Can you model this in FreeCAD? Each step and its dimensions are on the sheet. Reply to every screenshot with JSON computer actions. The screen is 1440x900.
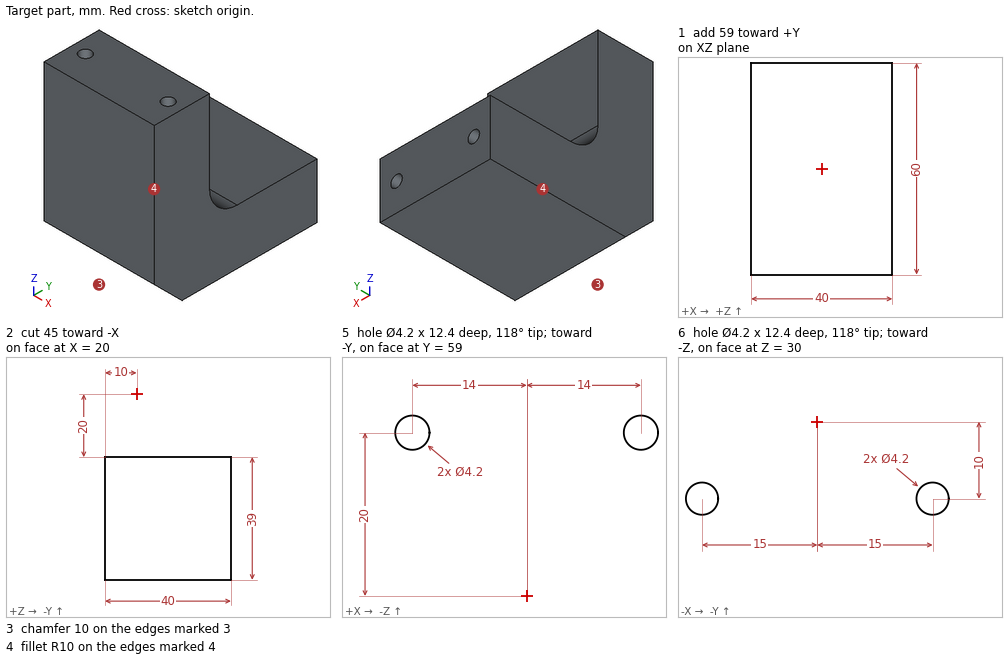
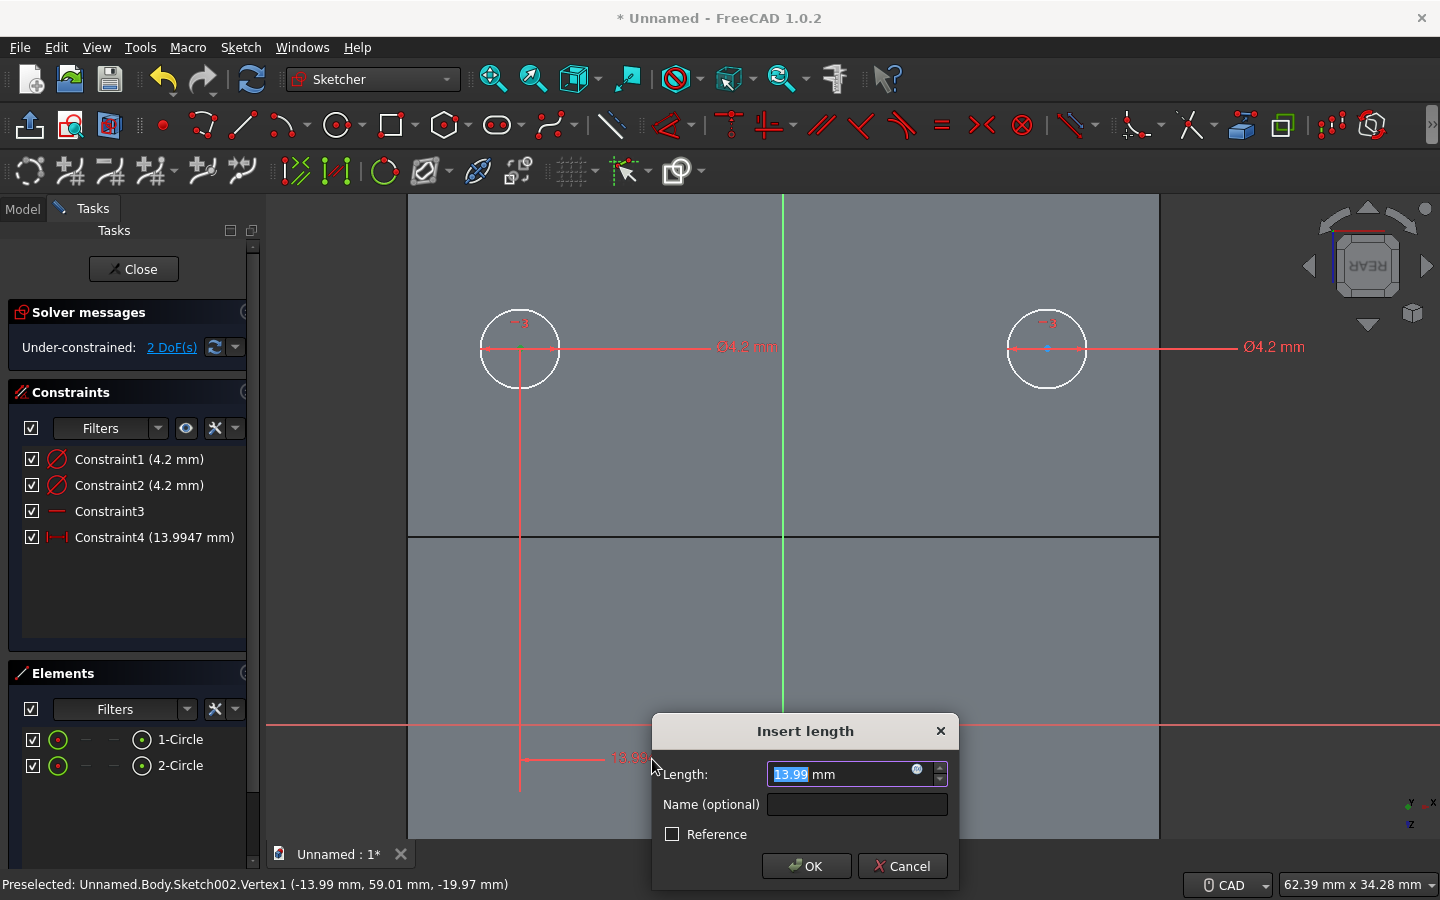
{"action": "type", "text": "14"}
{"action": "key", "text": "Return"}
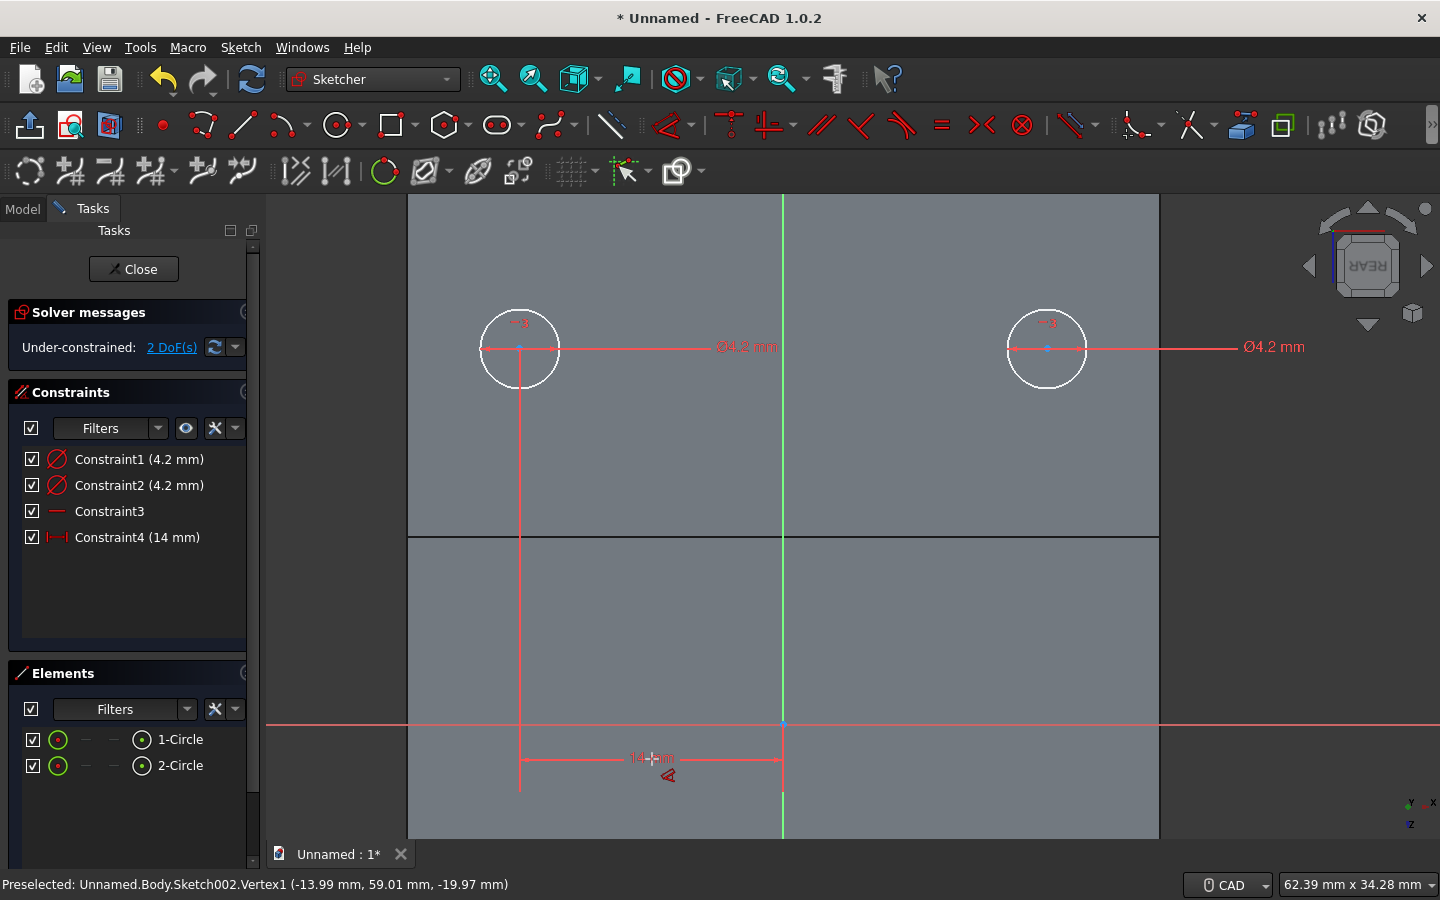
{"action": "left_click", "coordinate": [520, 349]}
{"action": "left_click", "coordinate": [486, 537]}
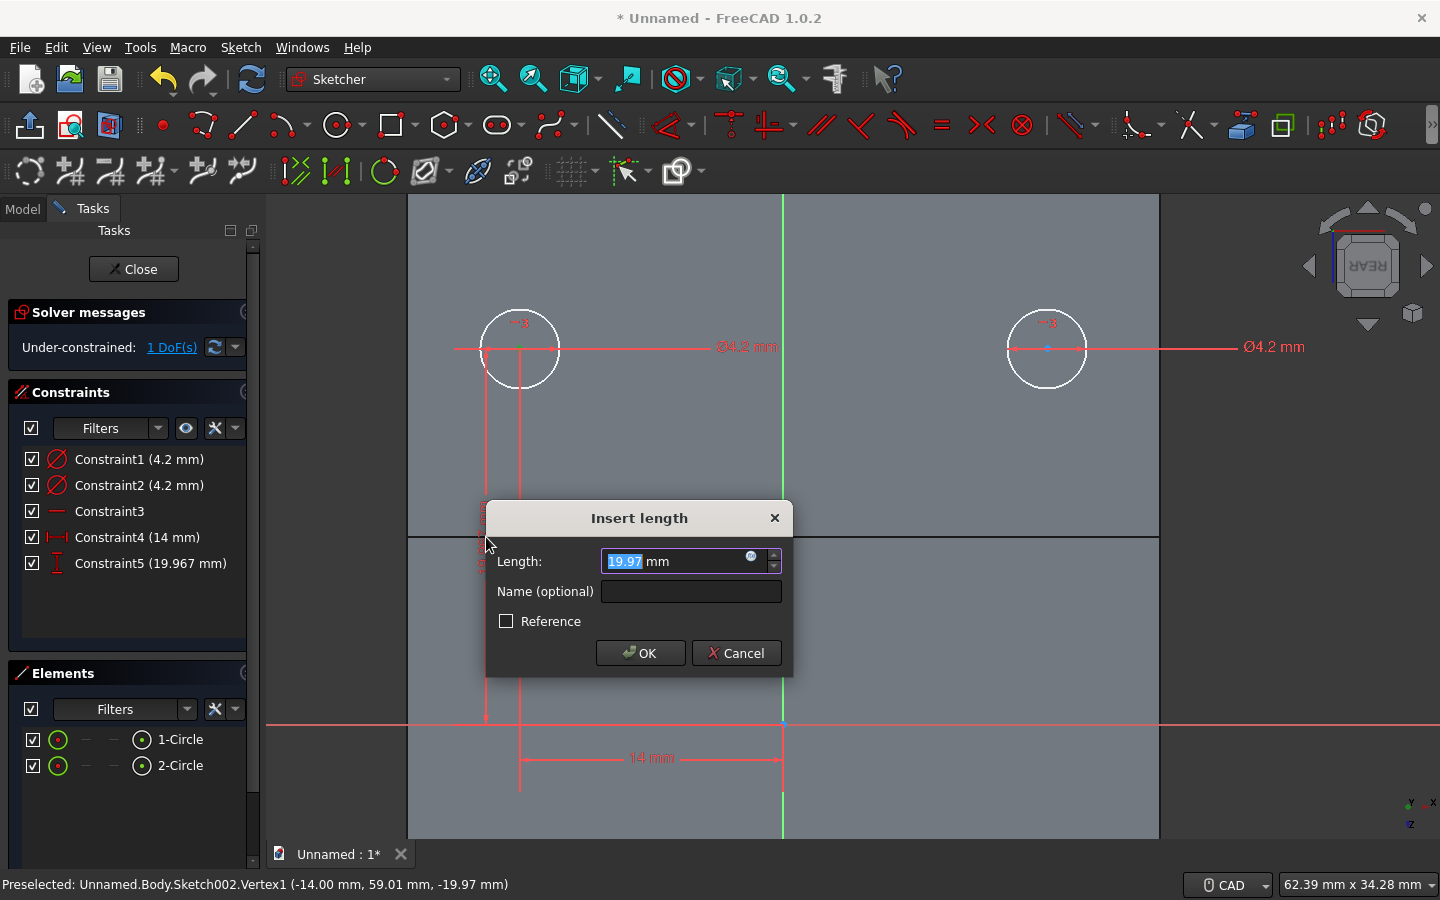
{"action": "type", "text": "20"}
{"action": "key", "text": "Return"}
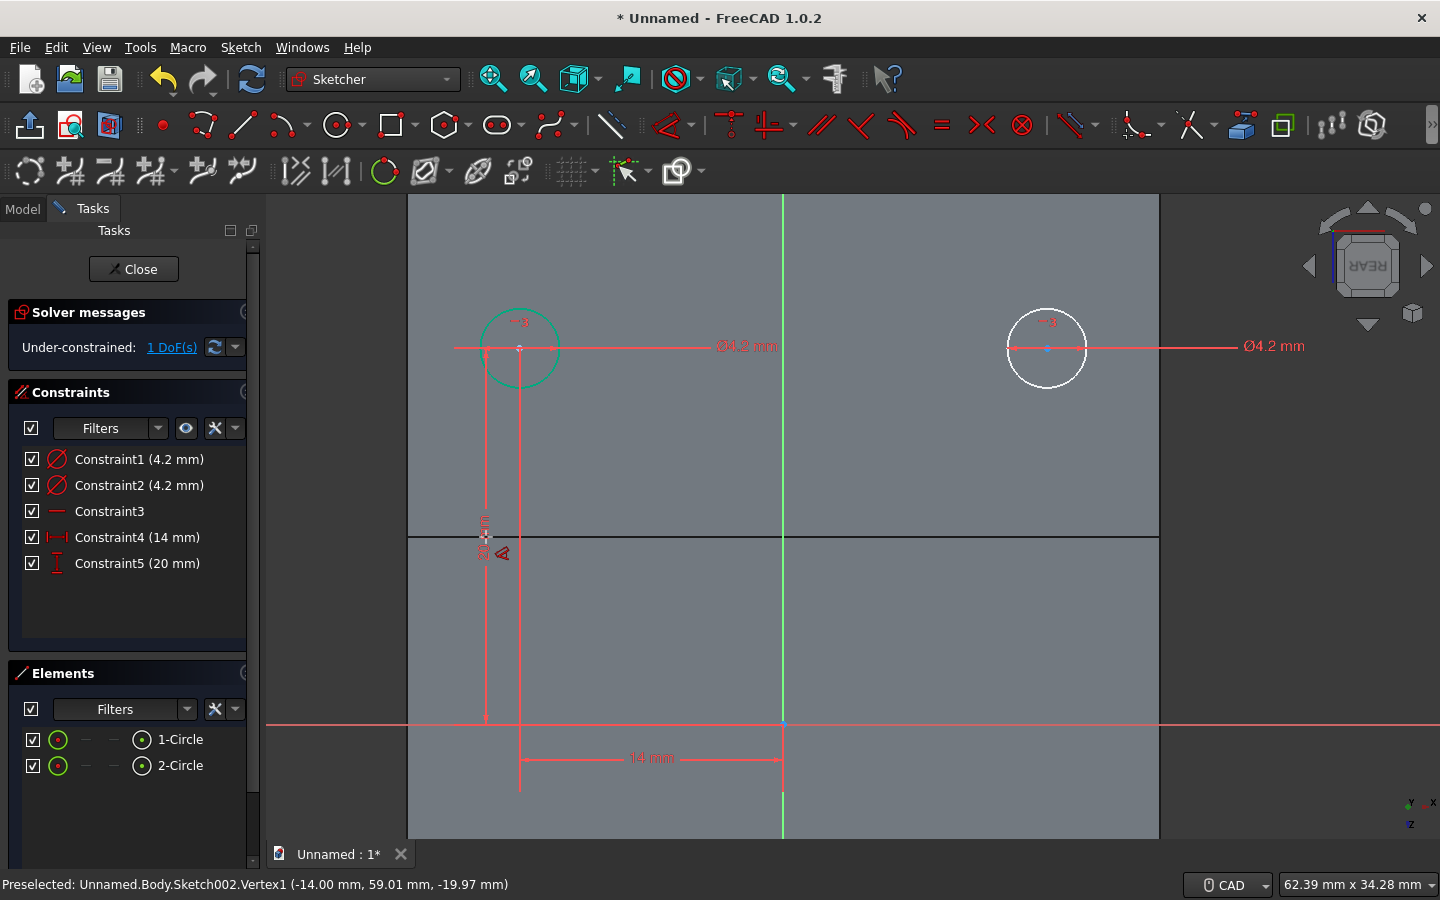
{"action": "left_click", "coordinate": [1047, 348]}
{"action": "left_click", "coordinate": [915, 759]}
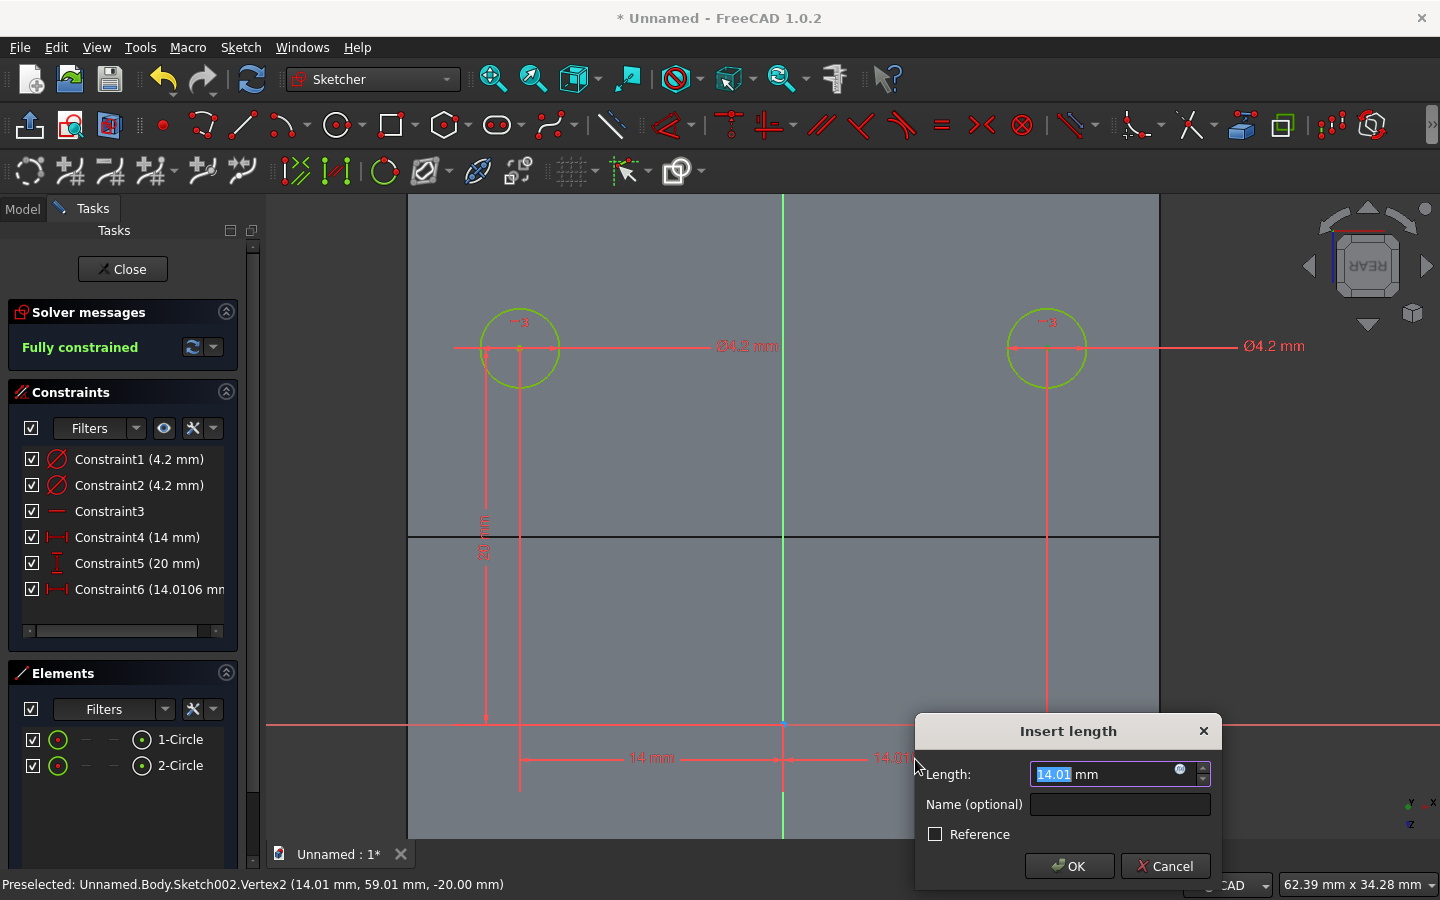
{"action": "type", "text": "14"}
{"action": "key", "text": "Return"}
{"action": "key", "text": "Escape"}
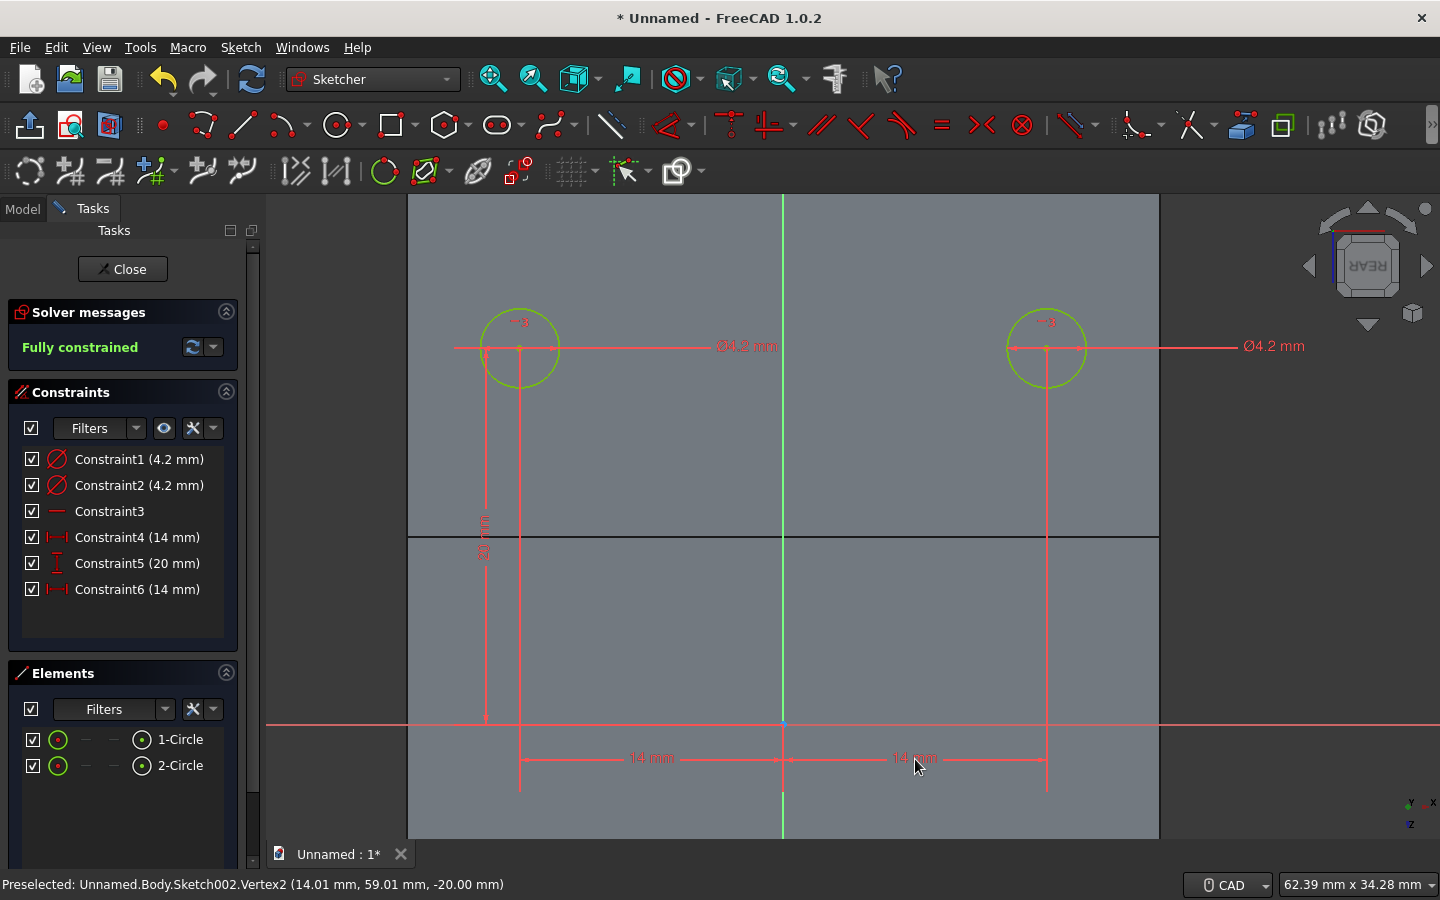
{"action": "left_click", "coordinate": [123, 269]}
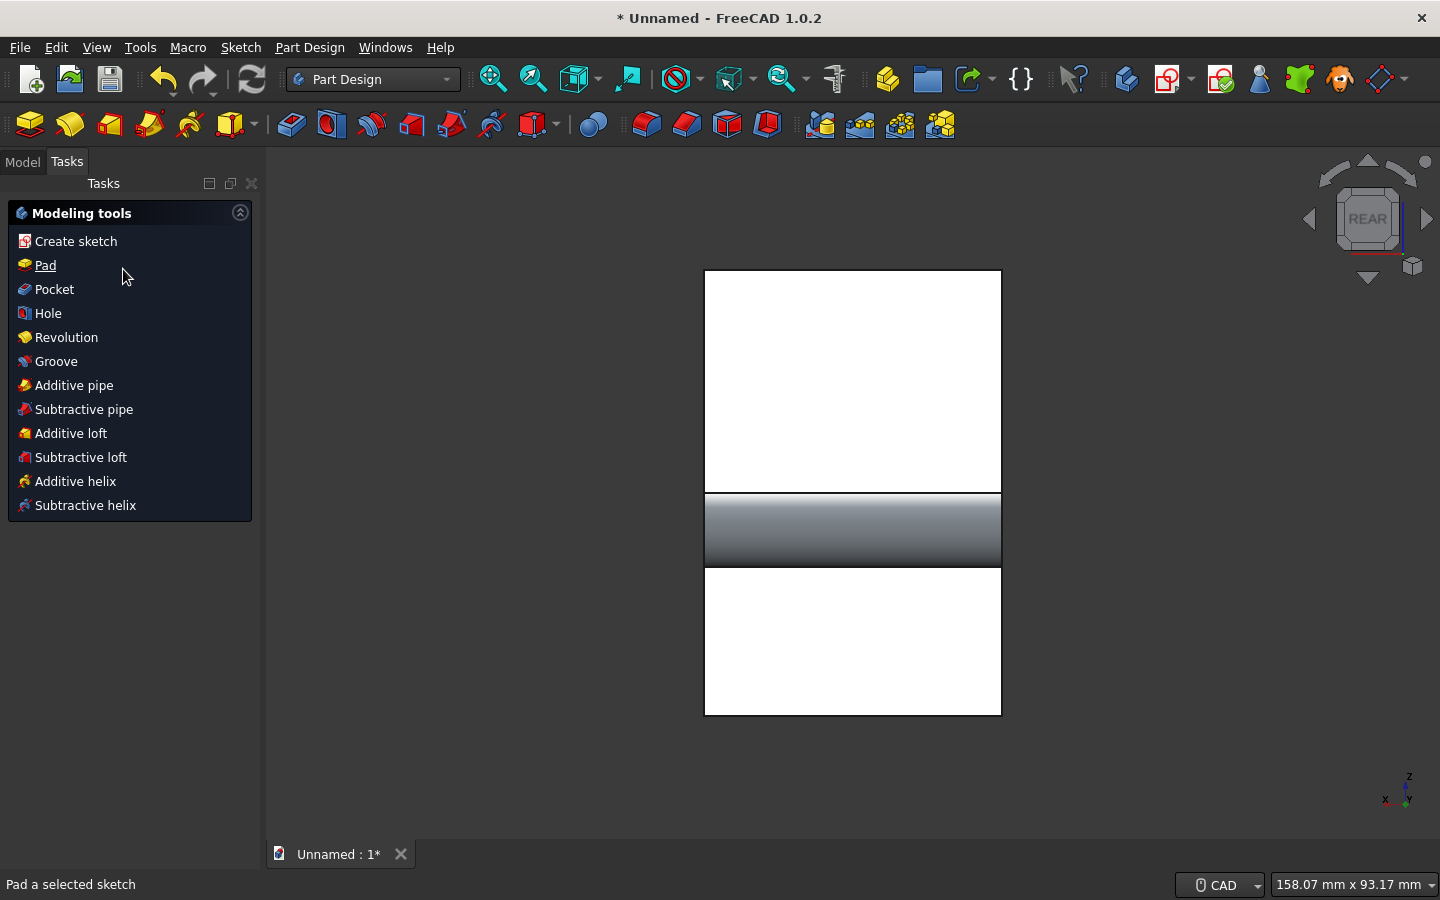
{"action": "left_click", "coordinate": [332, 124]}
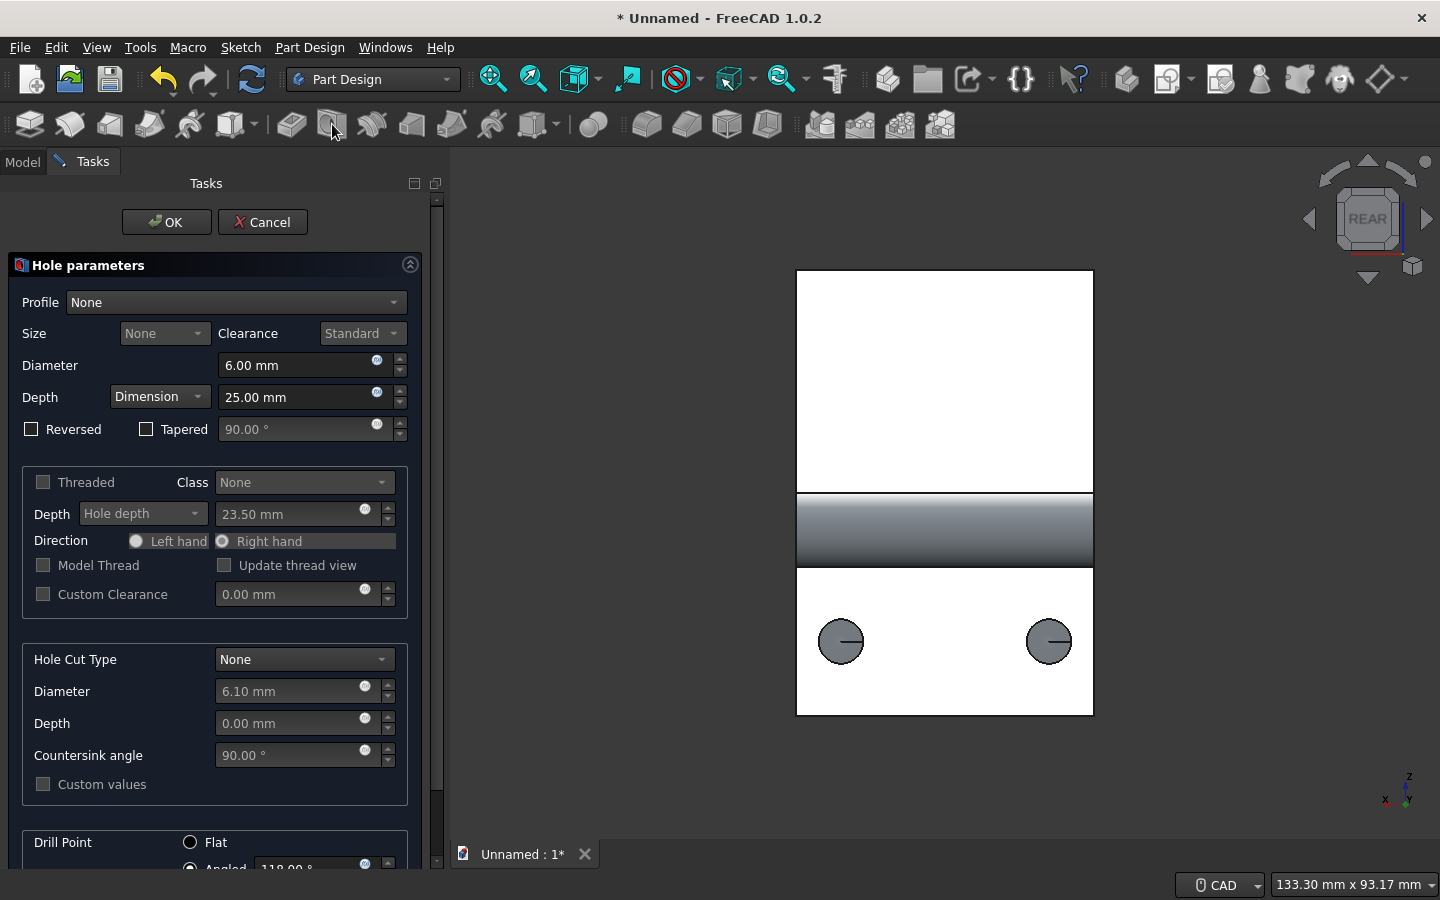
{"action": "triple_click", "coordinate": [305, 365]}